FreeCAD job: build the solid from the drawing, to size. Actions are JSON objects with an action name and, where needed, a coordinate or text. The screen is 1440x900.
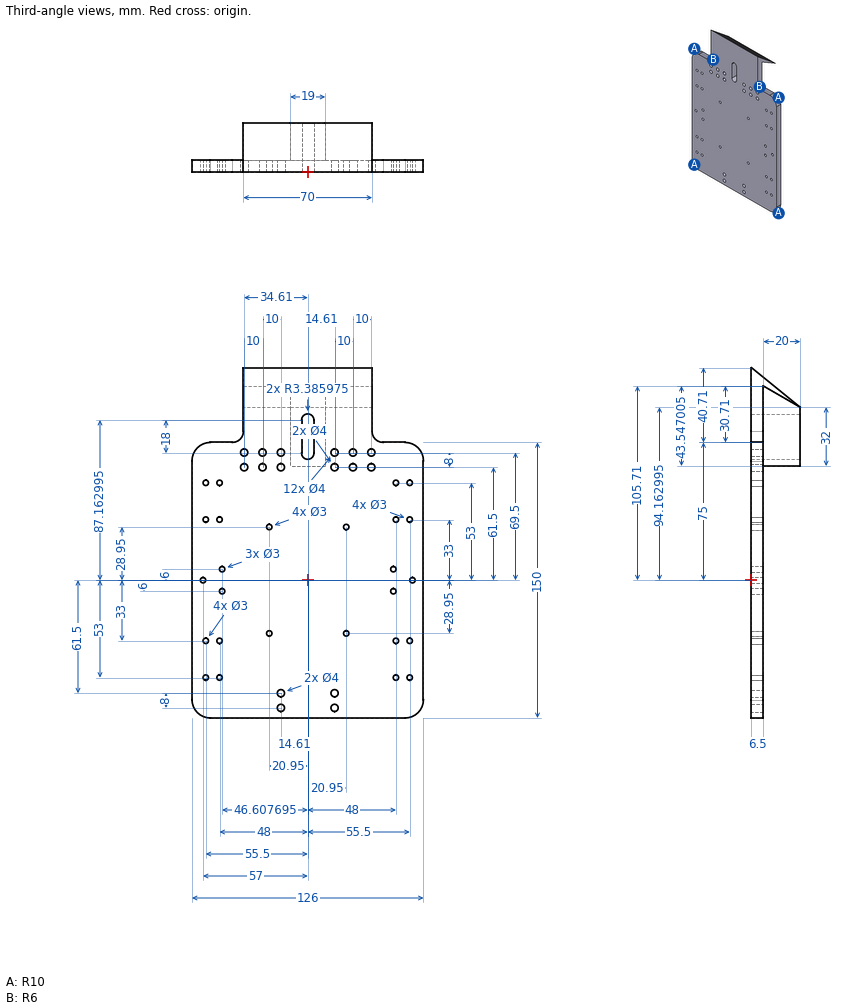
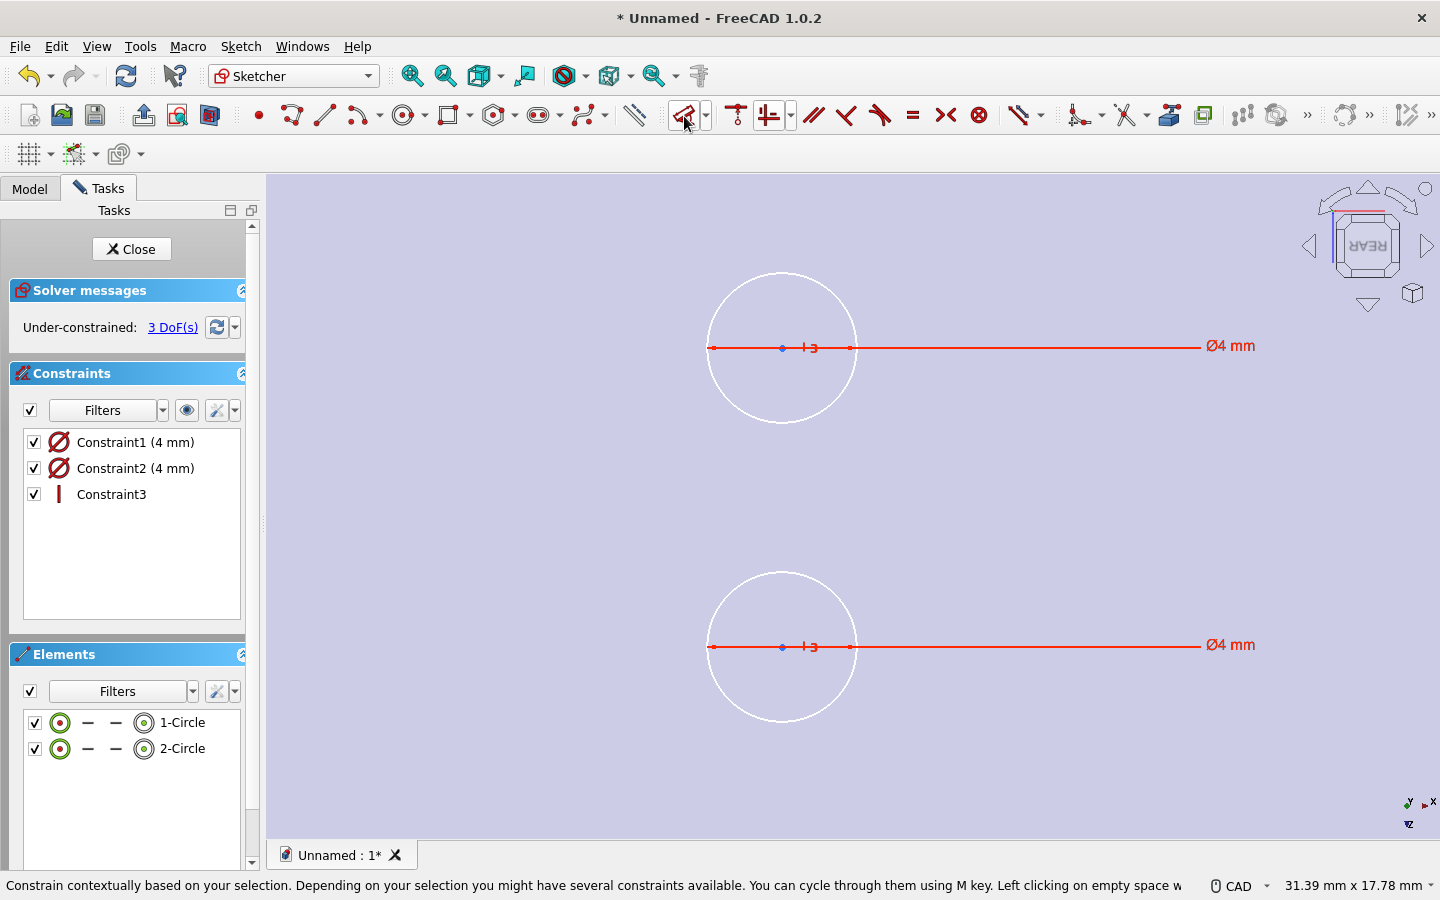
{"action": "left_click", "coordinate": [782, 348]}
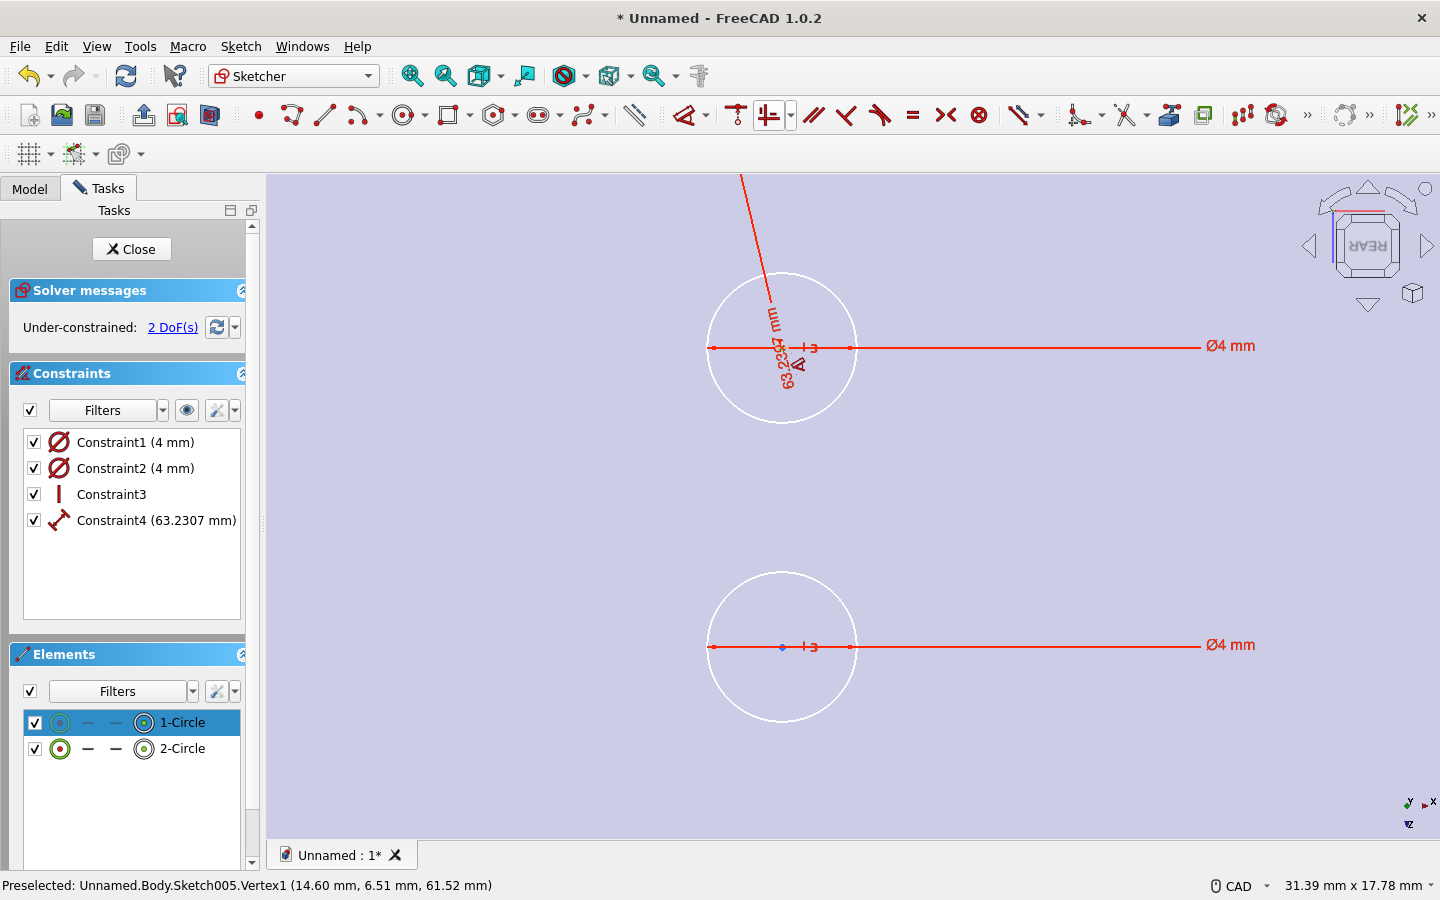
{"action": "left_click", "coordinate": [782, 647]}
{"action": "left_click", "coordinate": [748, 498]}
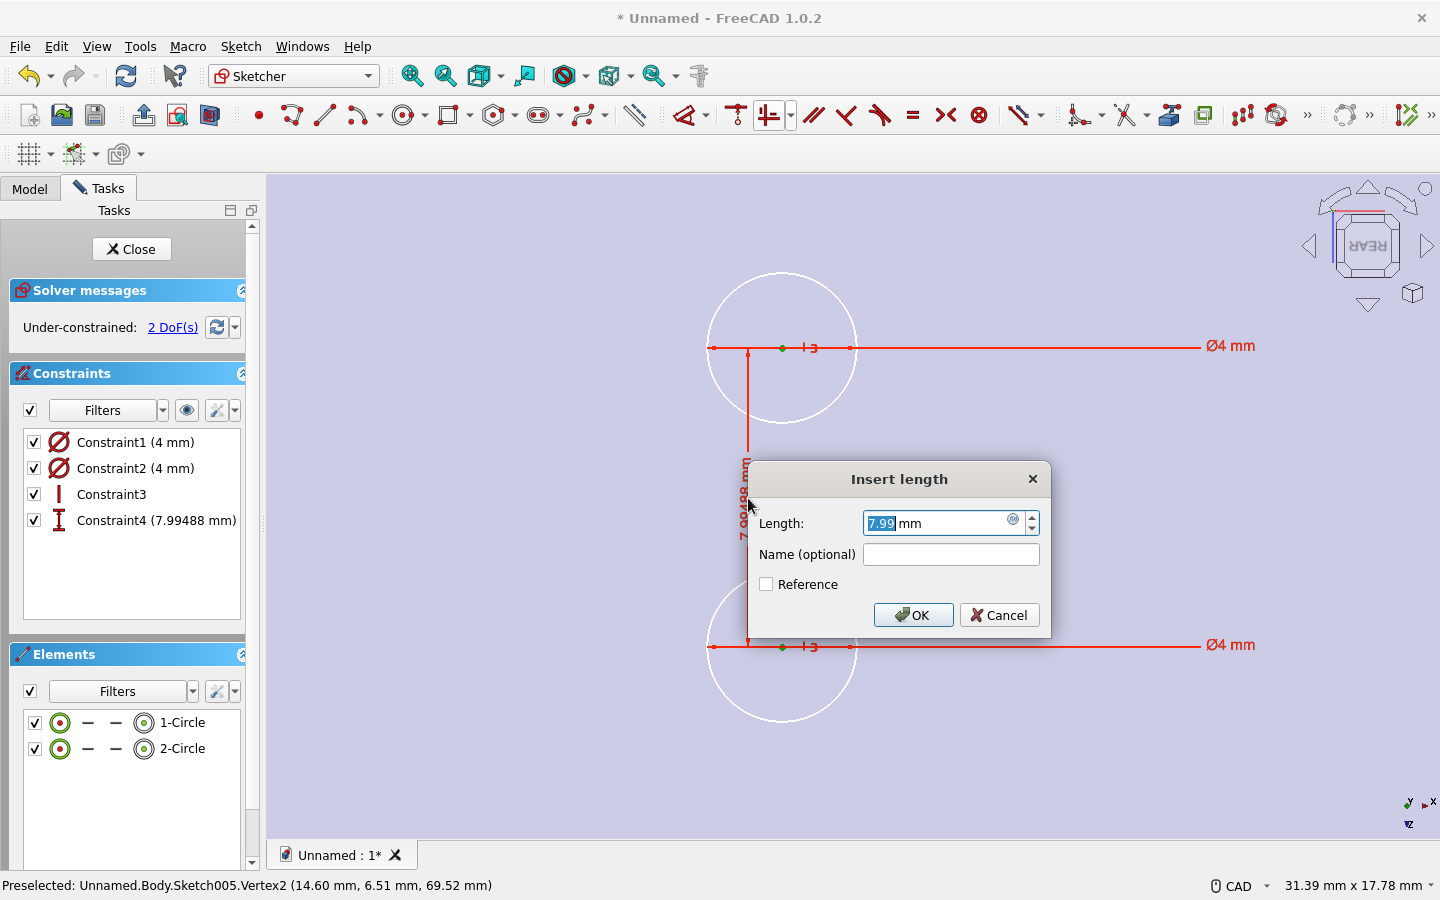
{"action": "type", "text": "8"}
{"action": "key", "text": "Return"}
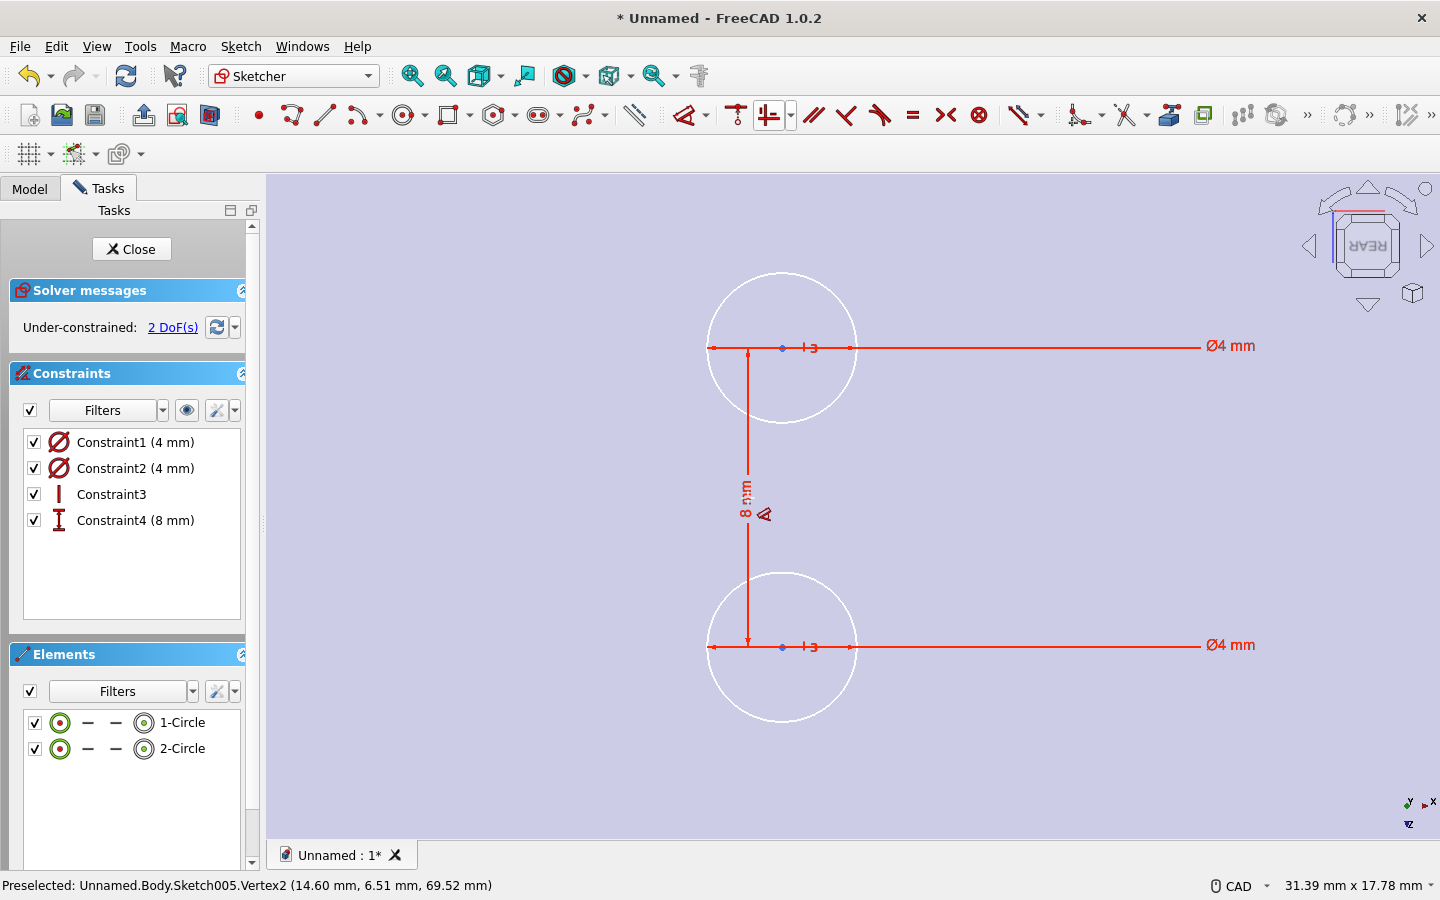
{"action": "left_click", "coordinate": [782, 348]}
{"action": "left_click", "coordinate": [816, 241]}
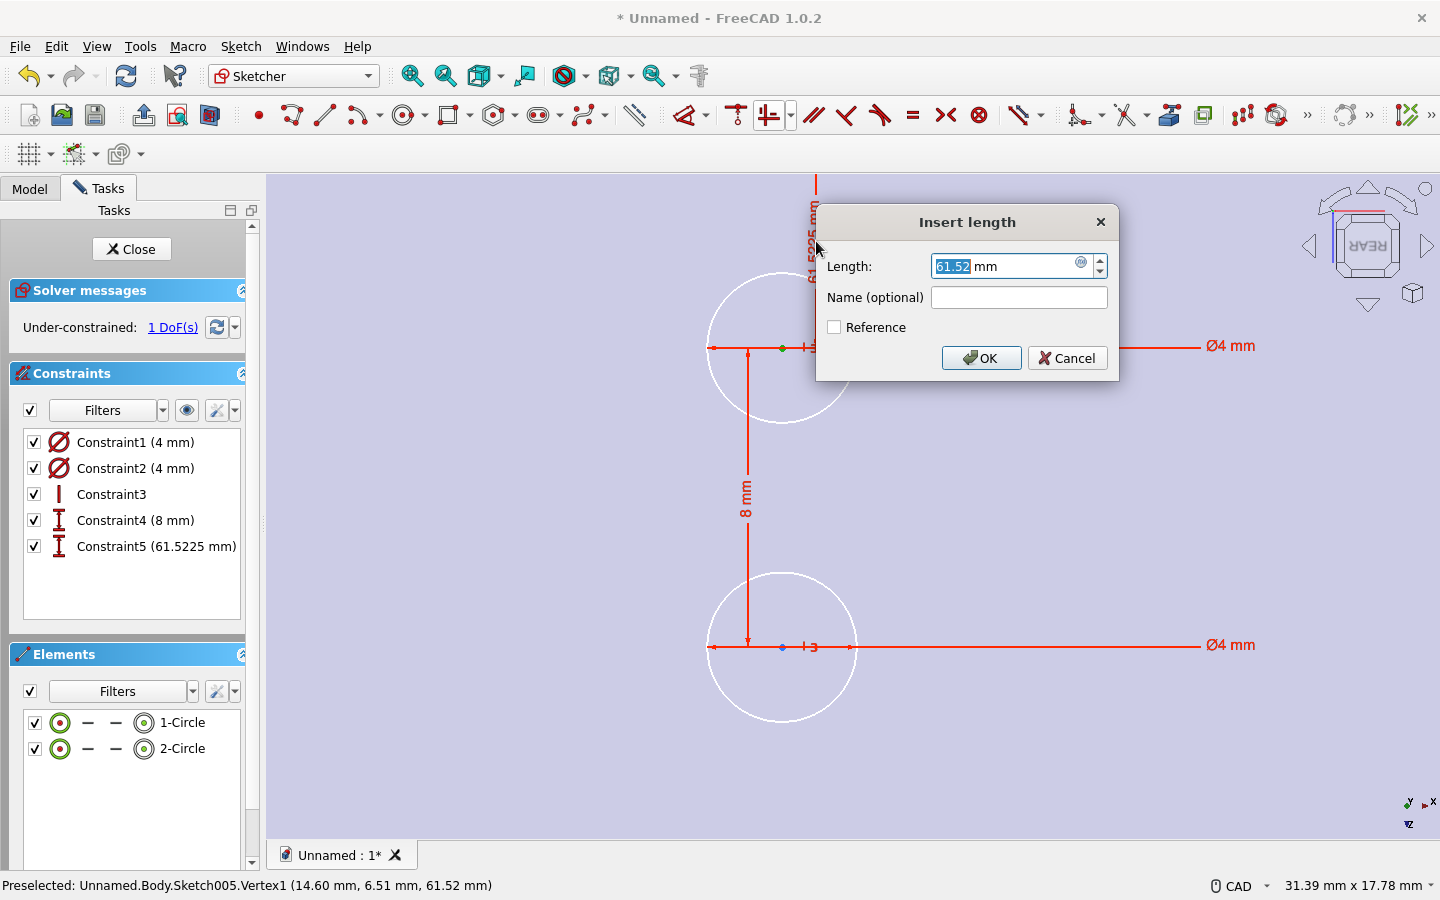
{"action": "type", "text": "61.5"}
{"action": "key", "text": "Return"}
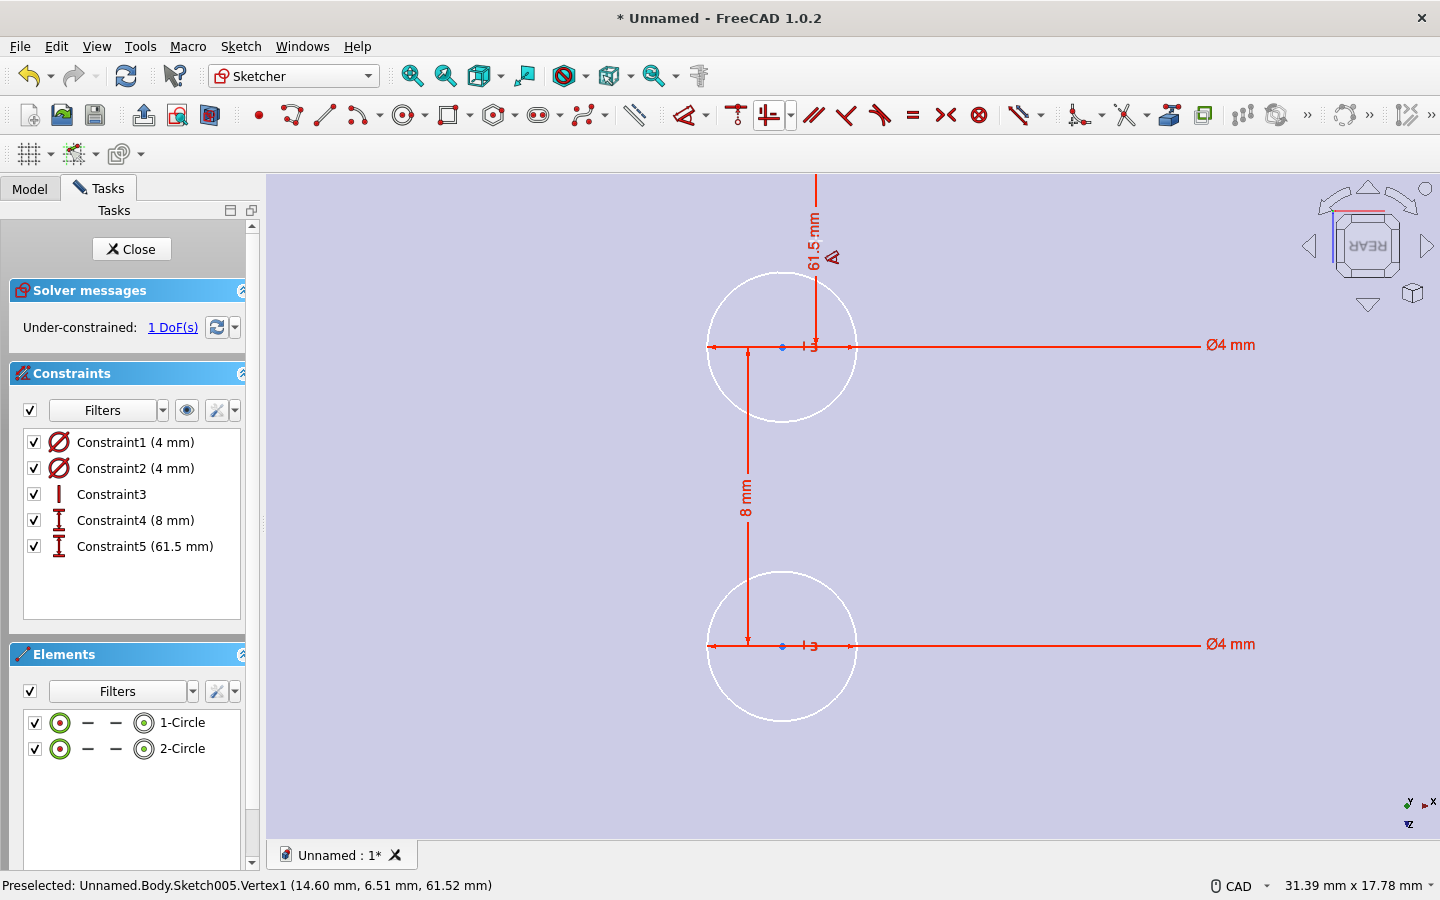
{"action": "left_click", "coordinate": [782, 347]}
{"action": "left_click", "coordinate": [538, 381]}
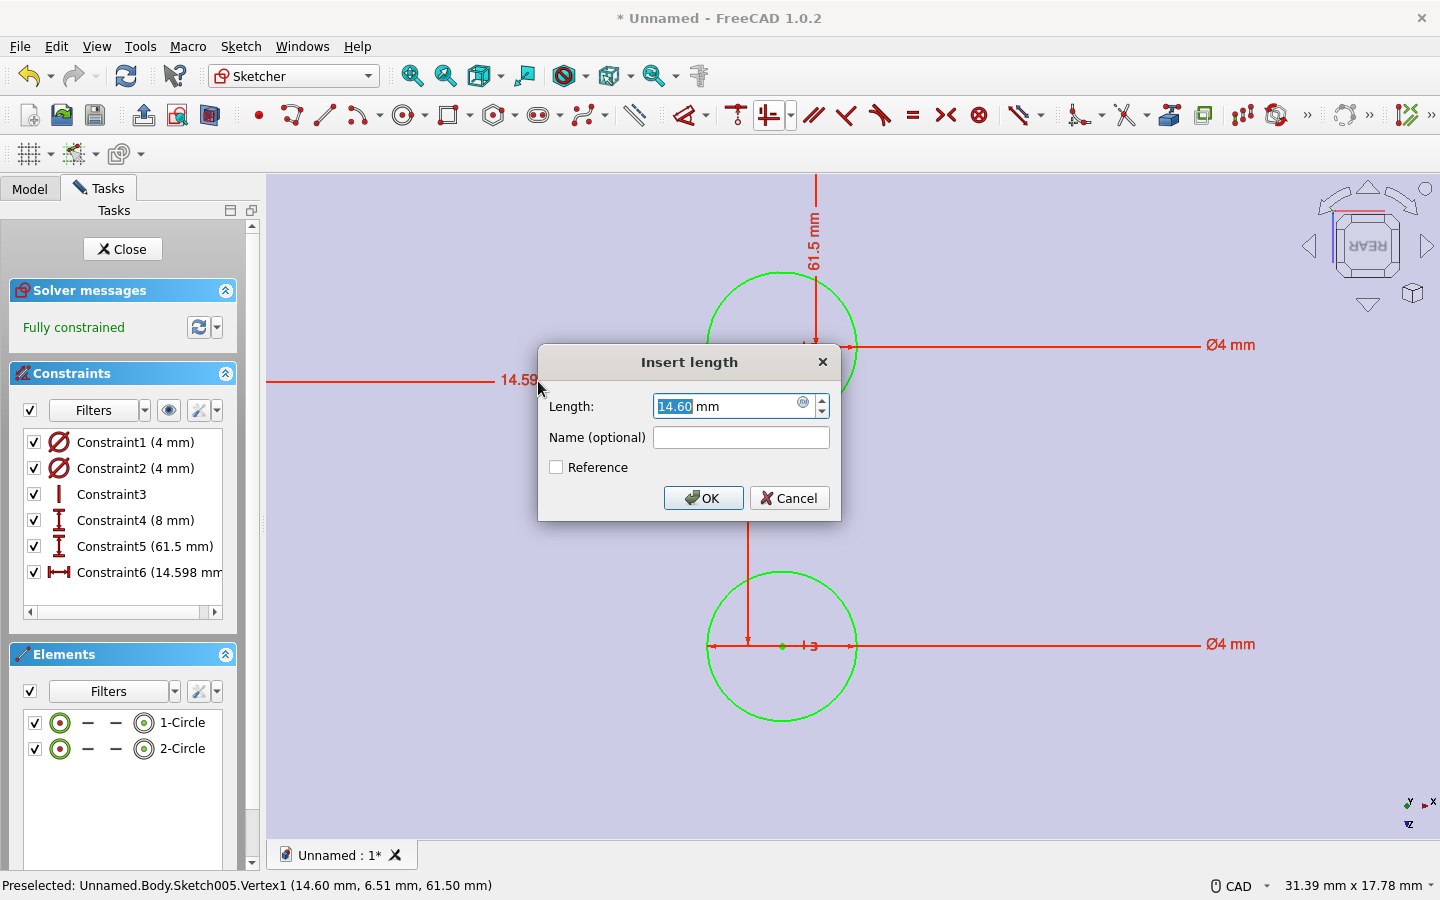
{"action": "type", "text": "14.61"}
{"action": "key", "text": "Return"}
{"action": "key", "text": "Escape"}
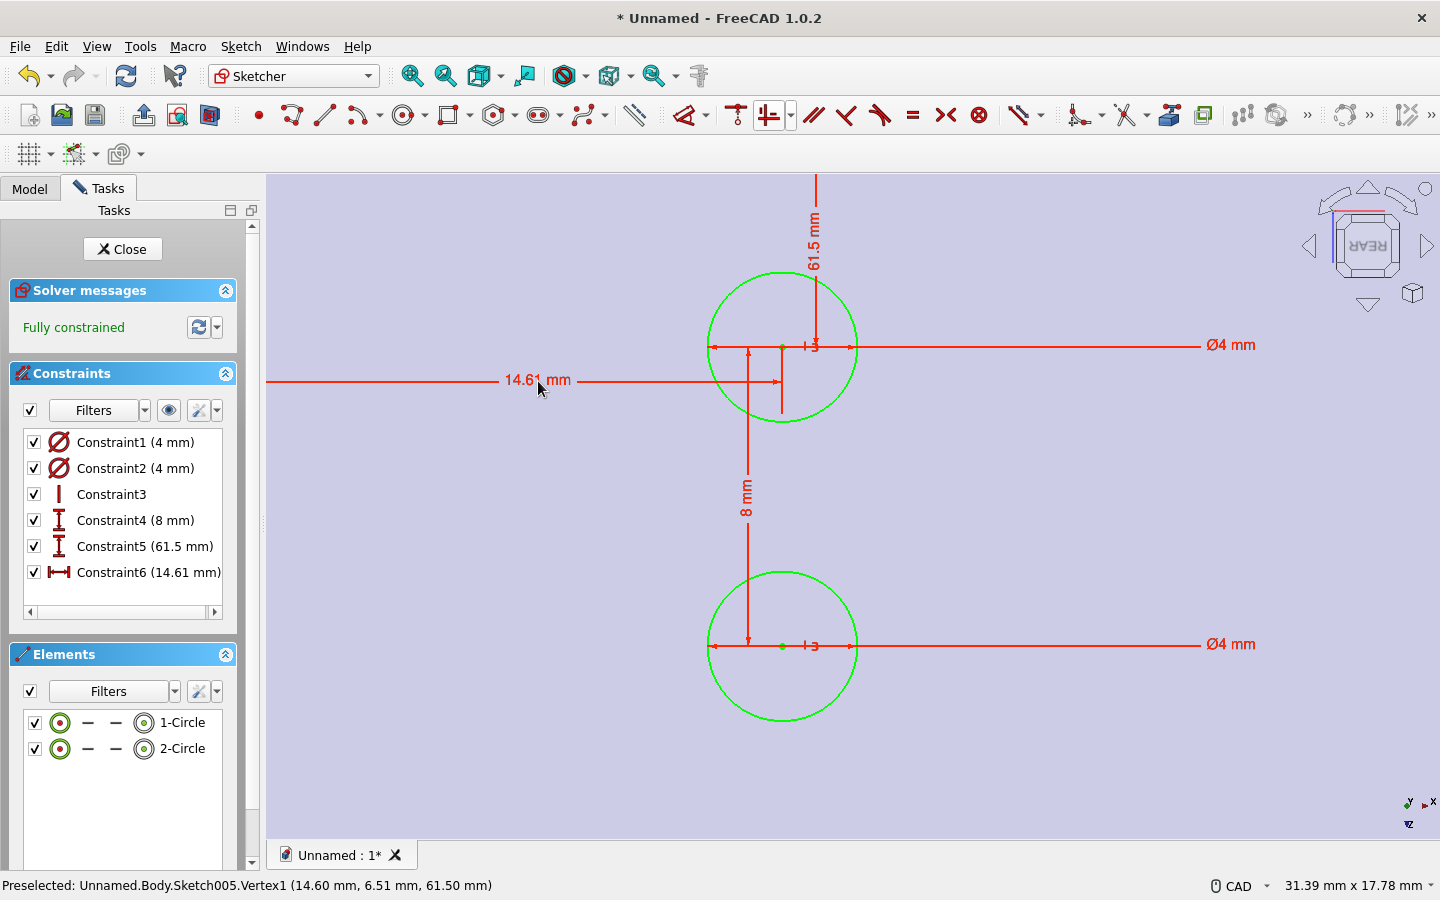
{"action": "left_click", "coordinate": [123, 249]}